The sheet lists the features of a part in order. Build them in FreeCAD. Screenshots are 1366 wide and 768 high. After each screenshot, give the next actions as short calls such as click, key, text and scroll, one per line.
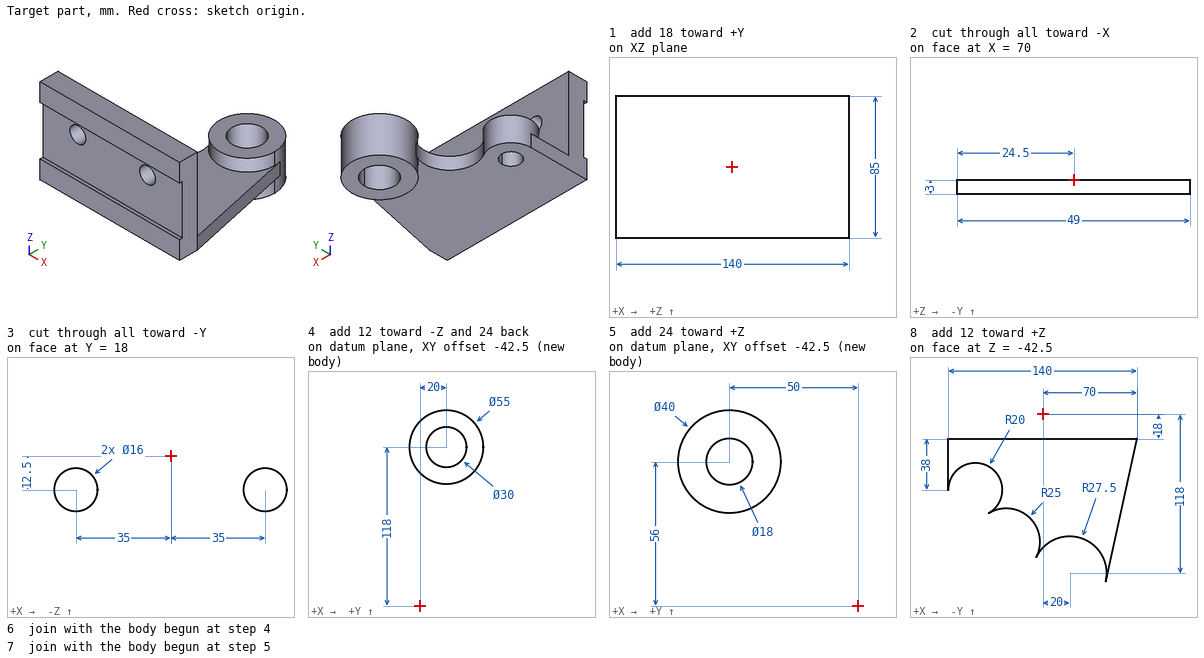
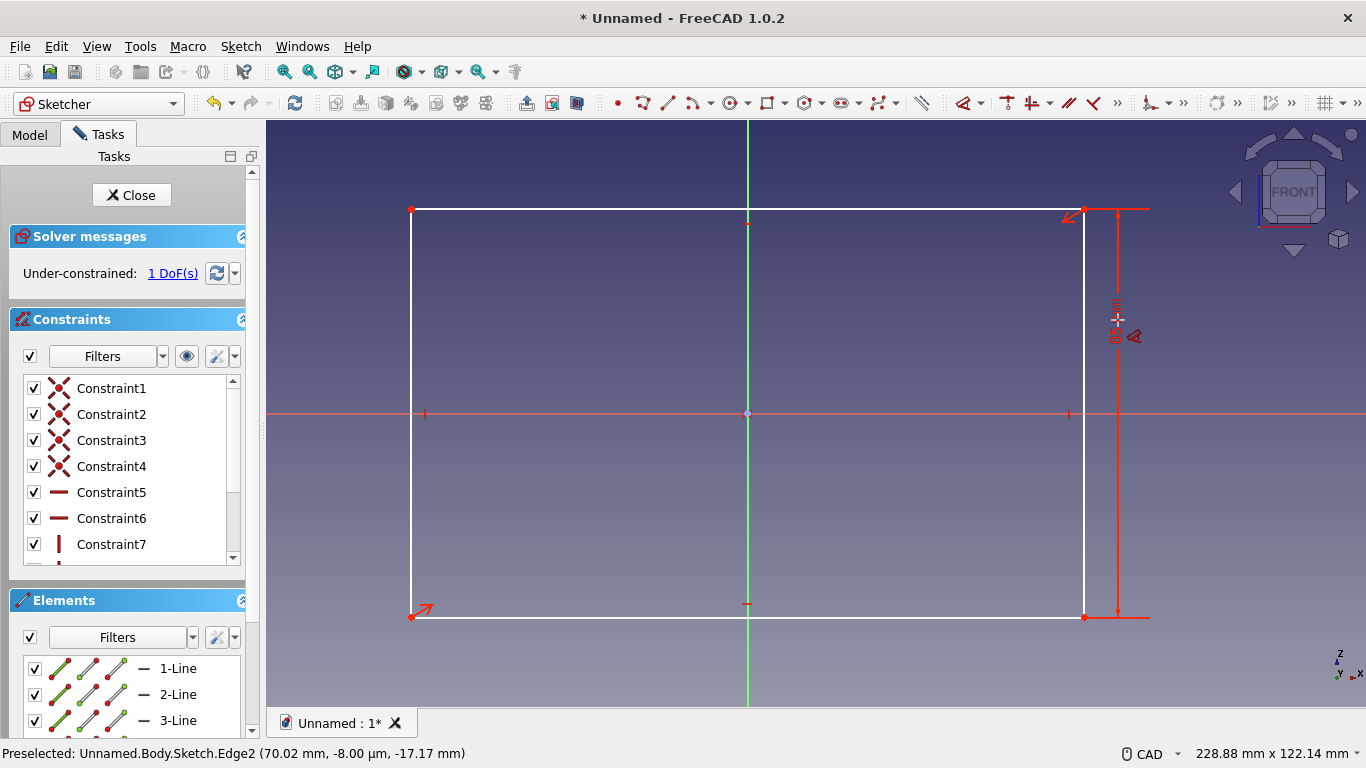
click(613, 618)
click(593, 652)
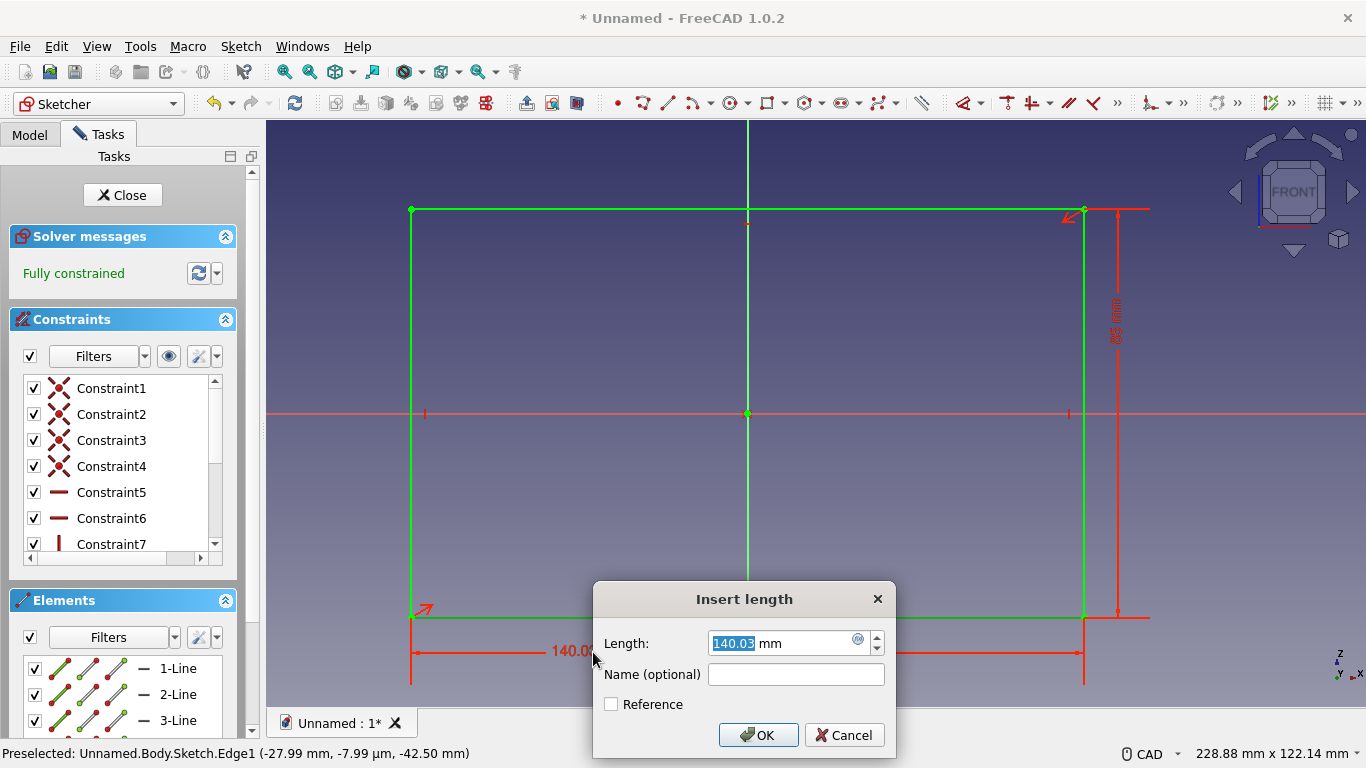
text(140)
key(Return)
key(Escape)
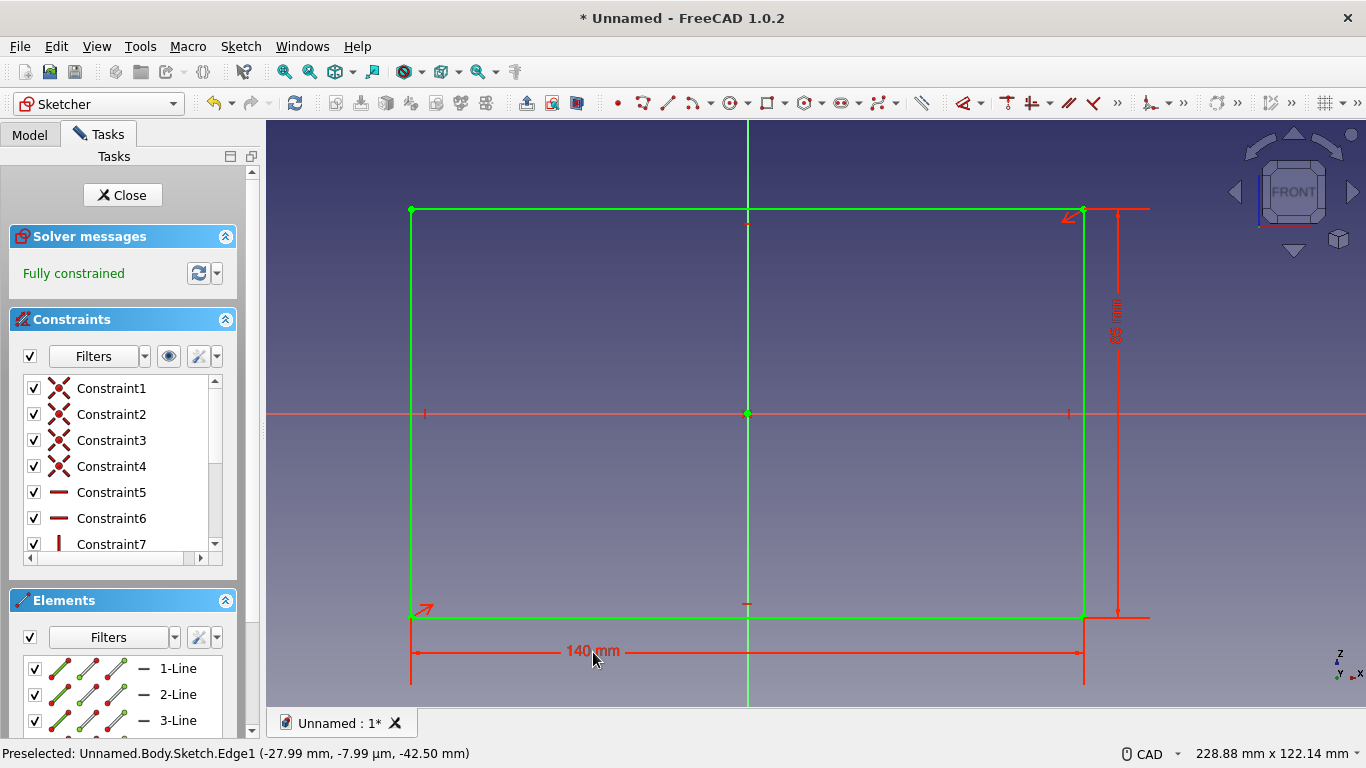
click(123, 195)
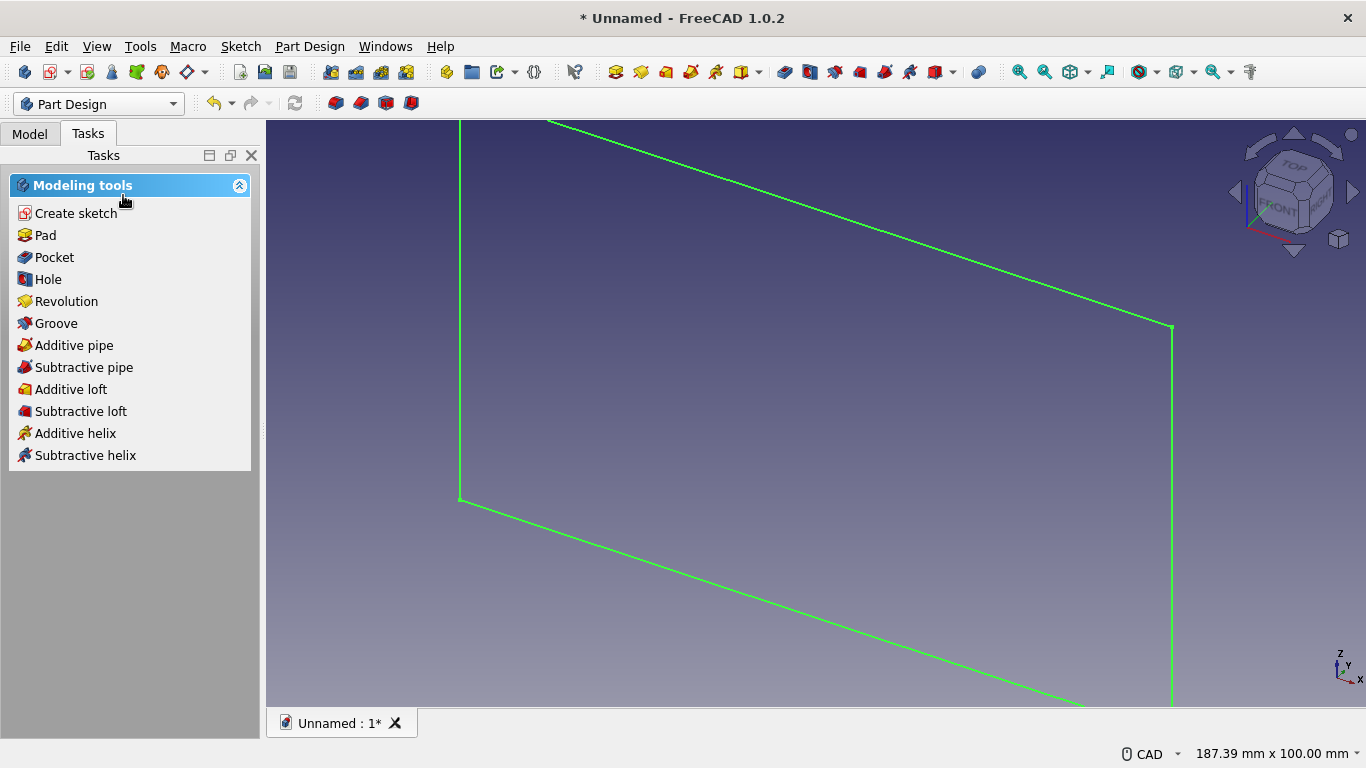
click(616, 72)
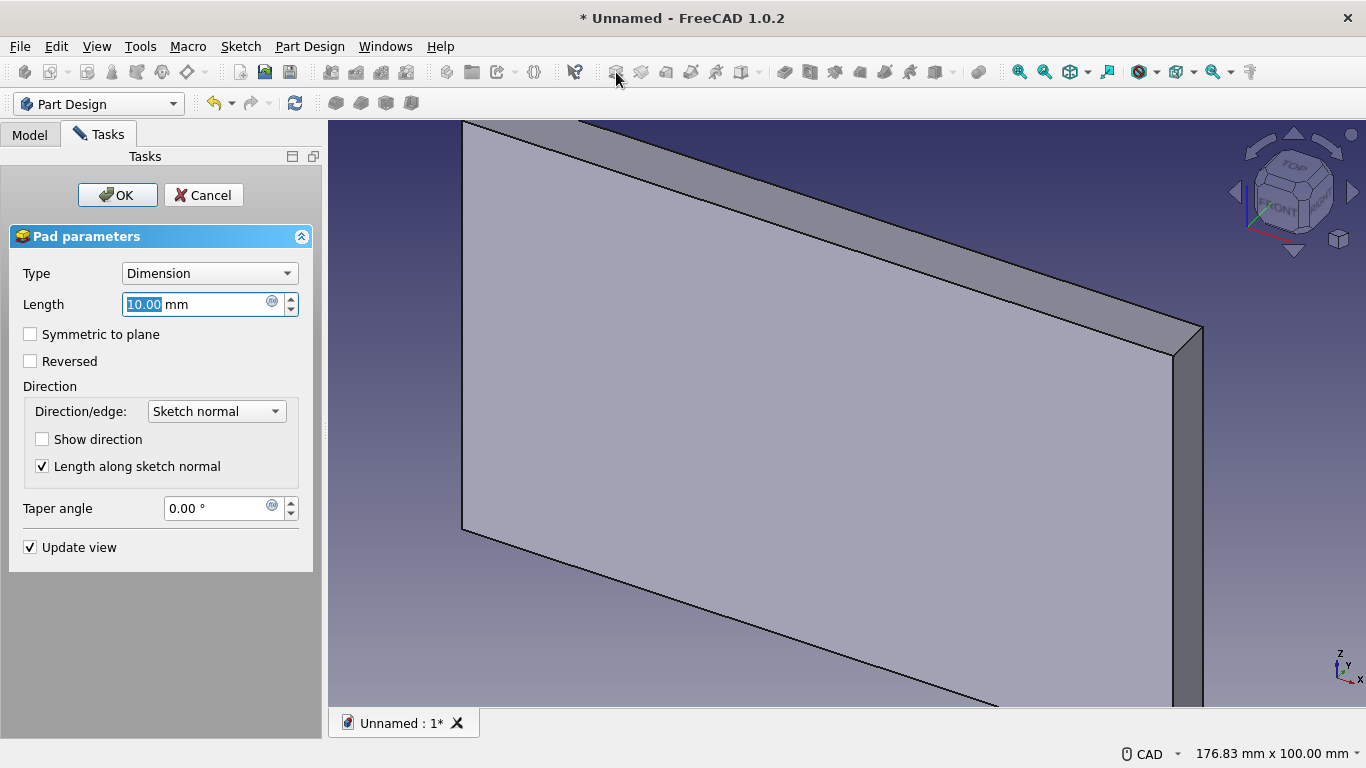
text(18)
key(Tab)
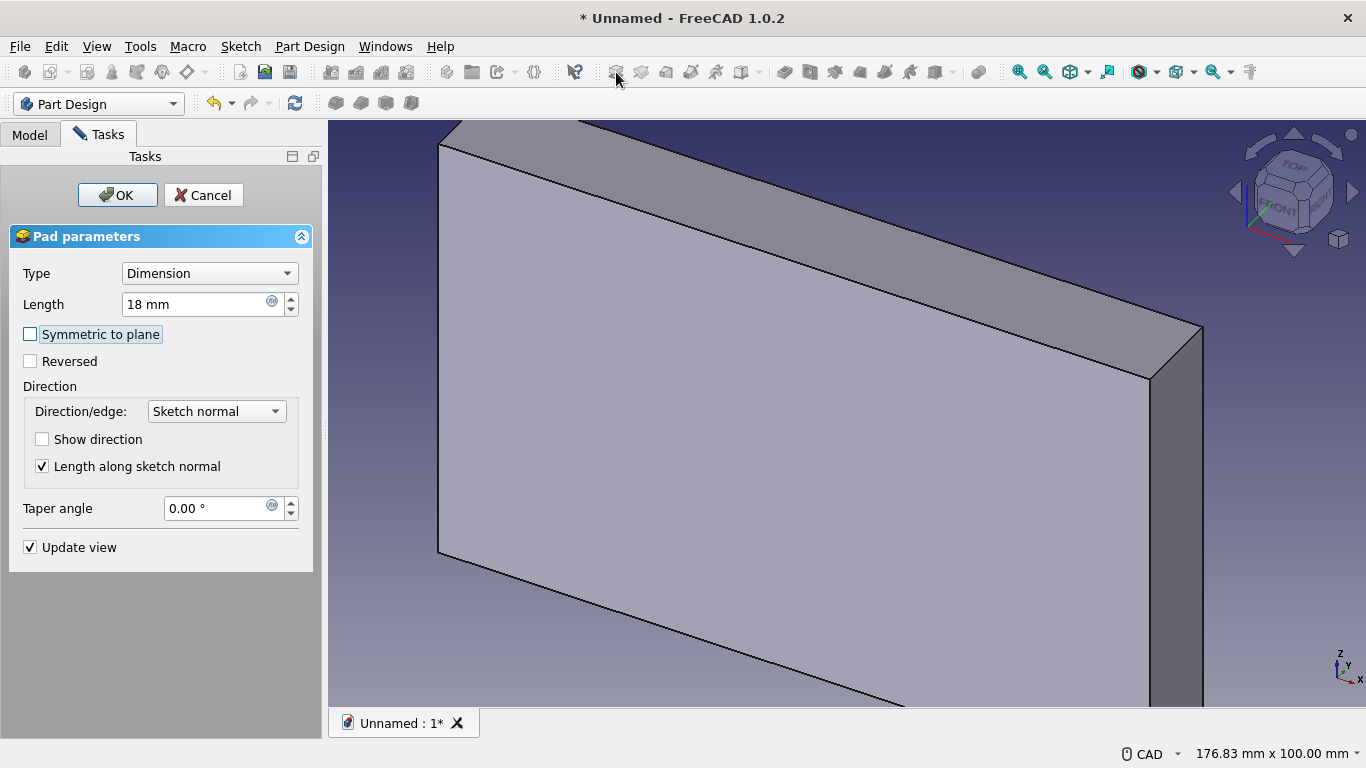
click(31, 361)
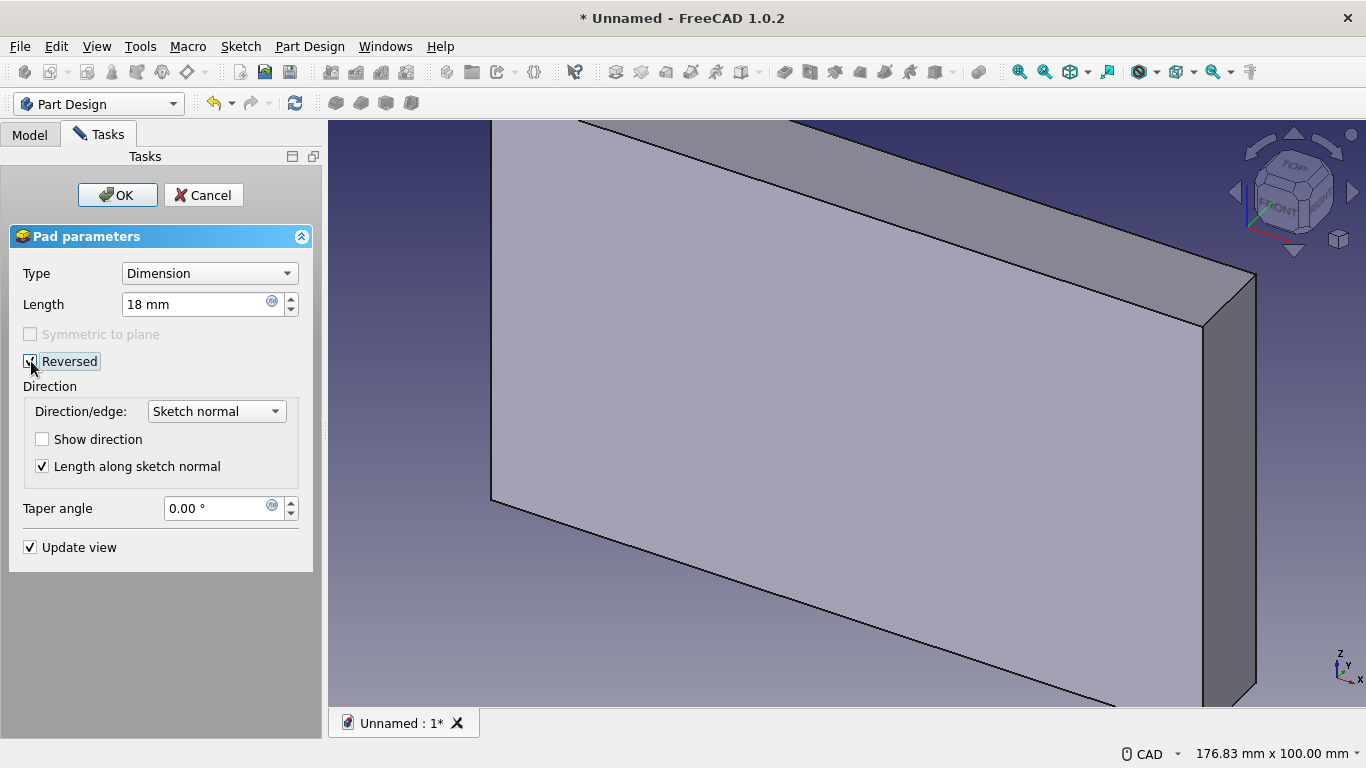
click(118, 195)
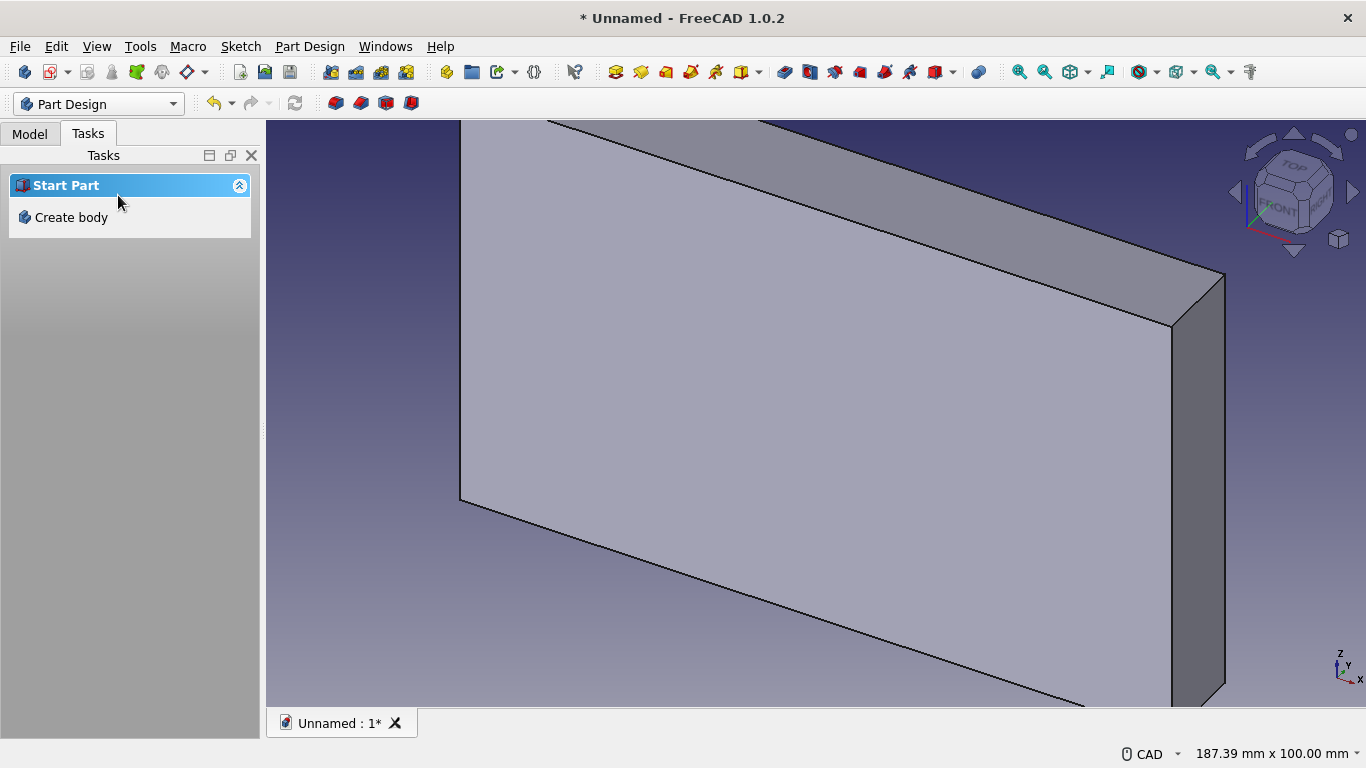
click(1020, 72)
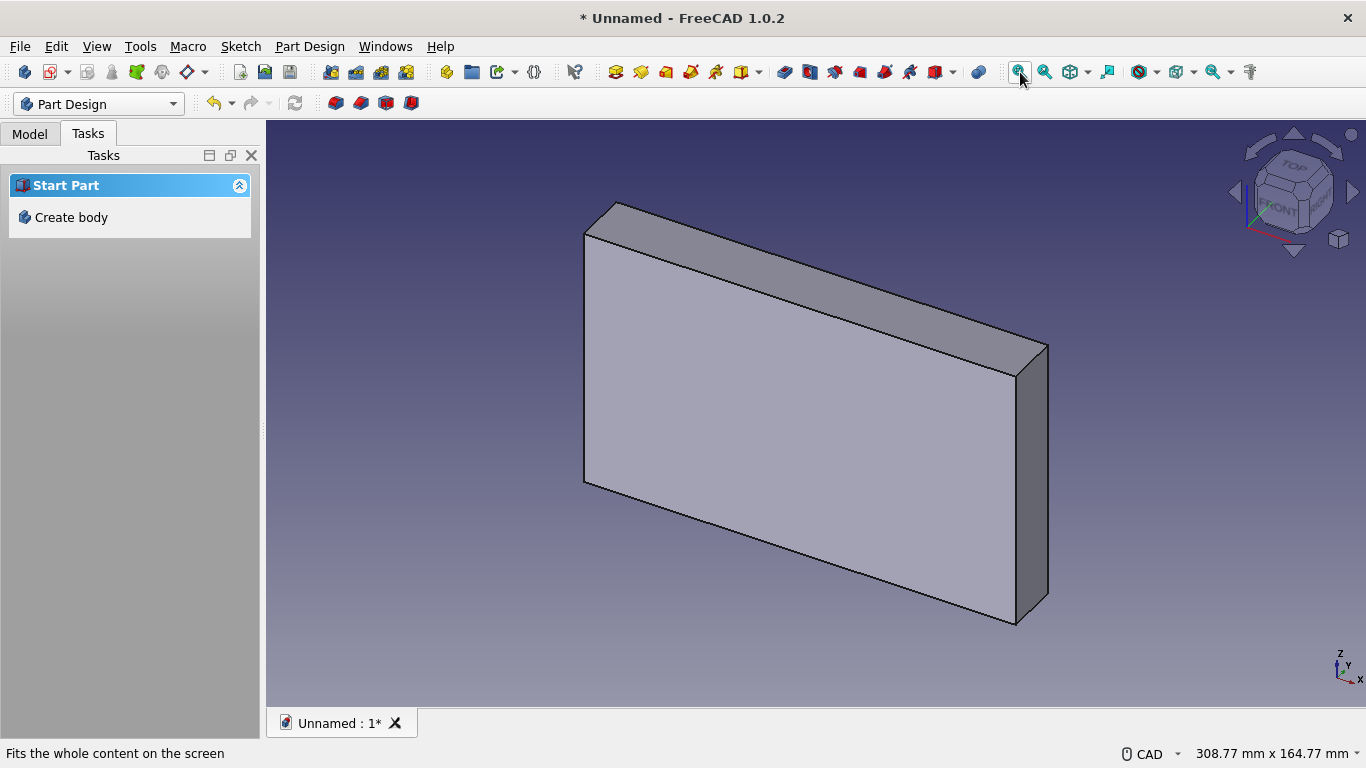
click(1032, 484)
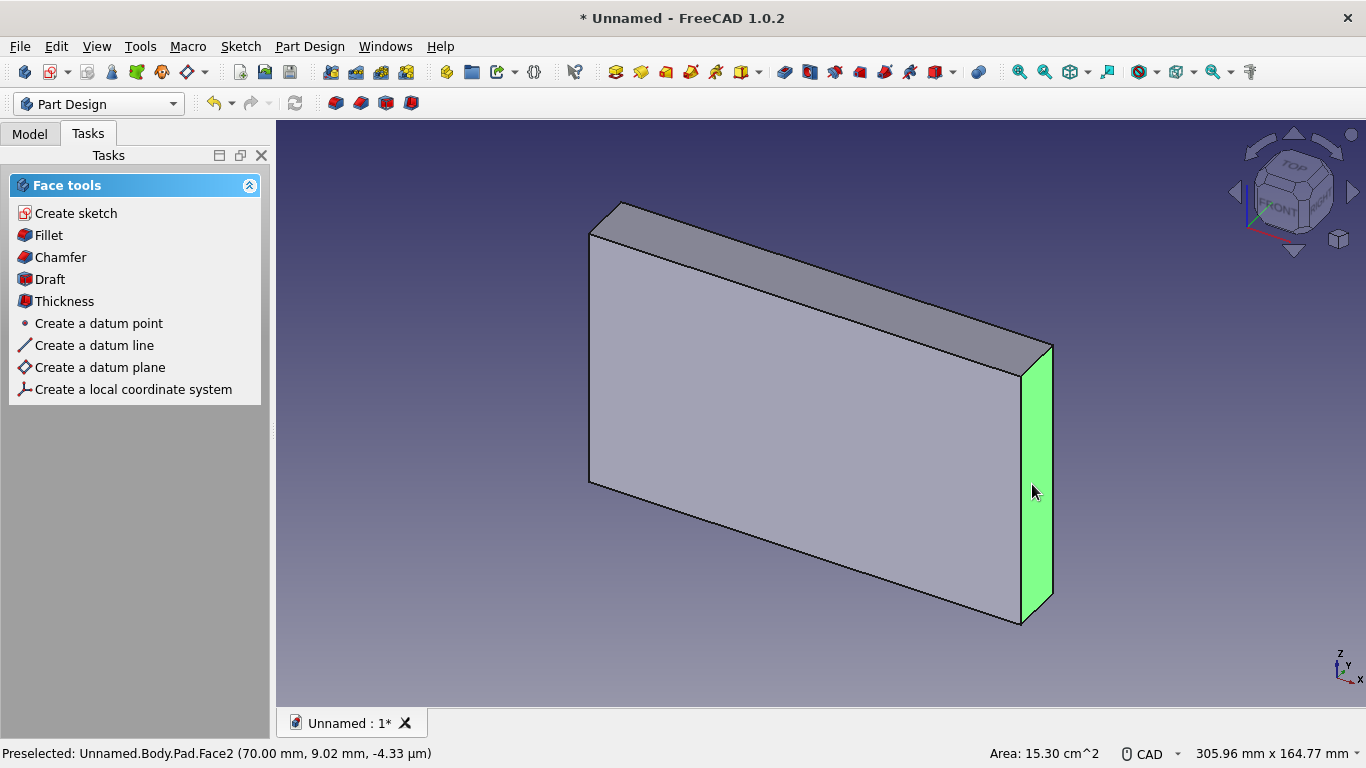
click(50, 72)